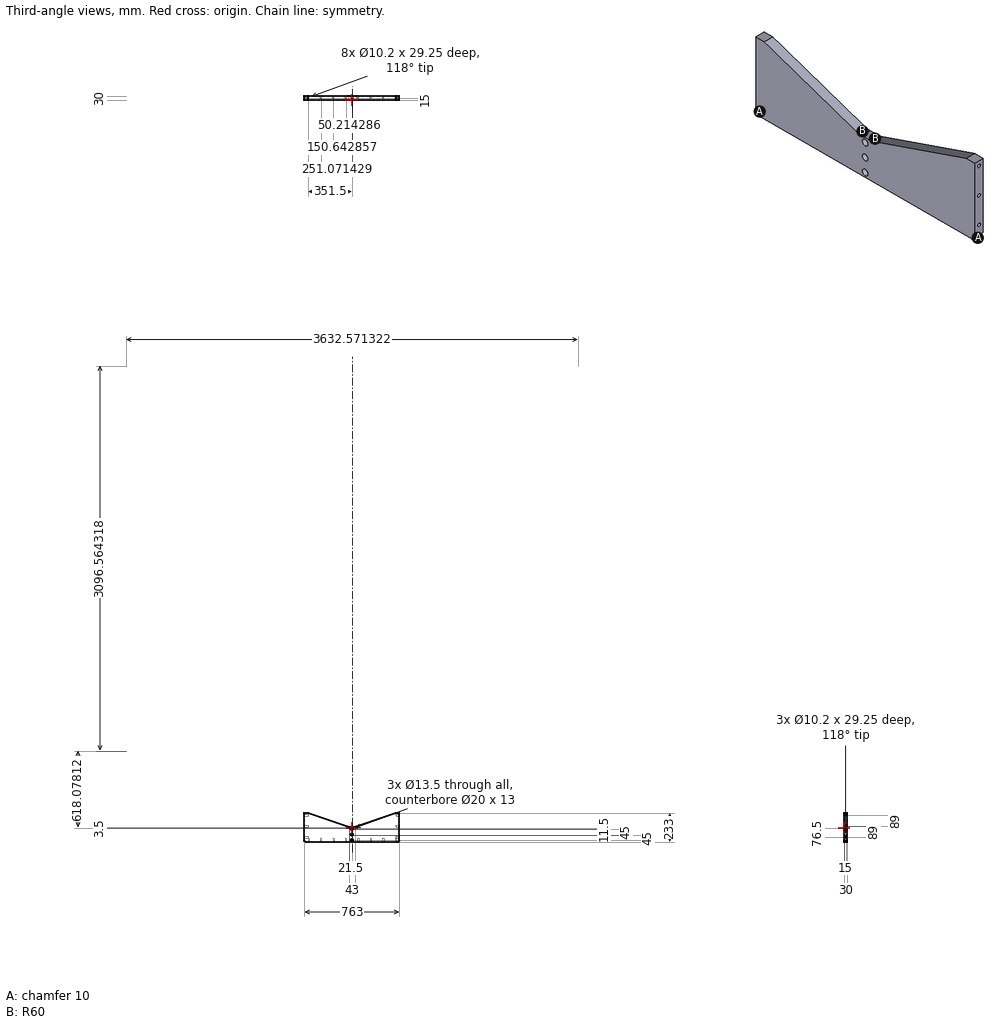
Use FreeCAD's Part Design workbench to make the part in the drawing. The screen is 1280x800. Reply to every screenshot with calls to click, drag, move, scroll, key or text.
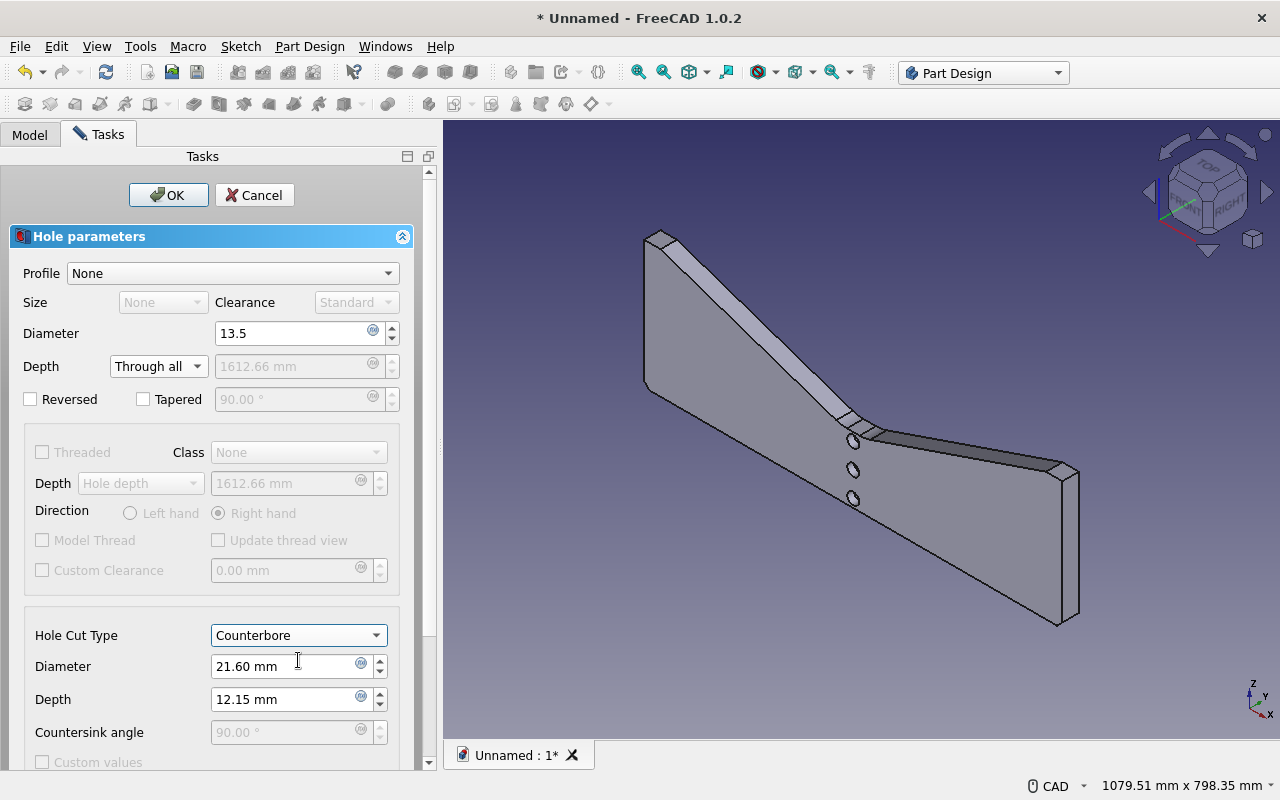
triple_click(292, 666)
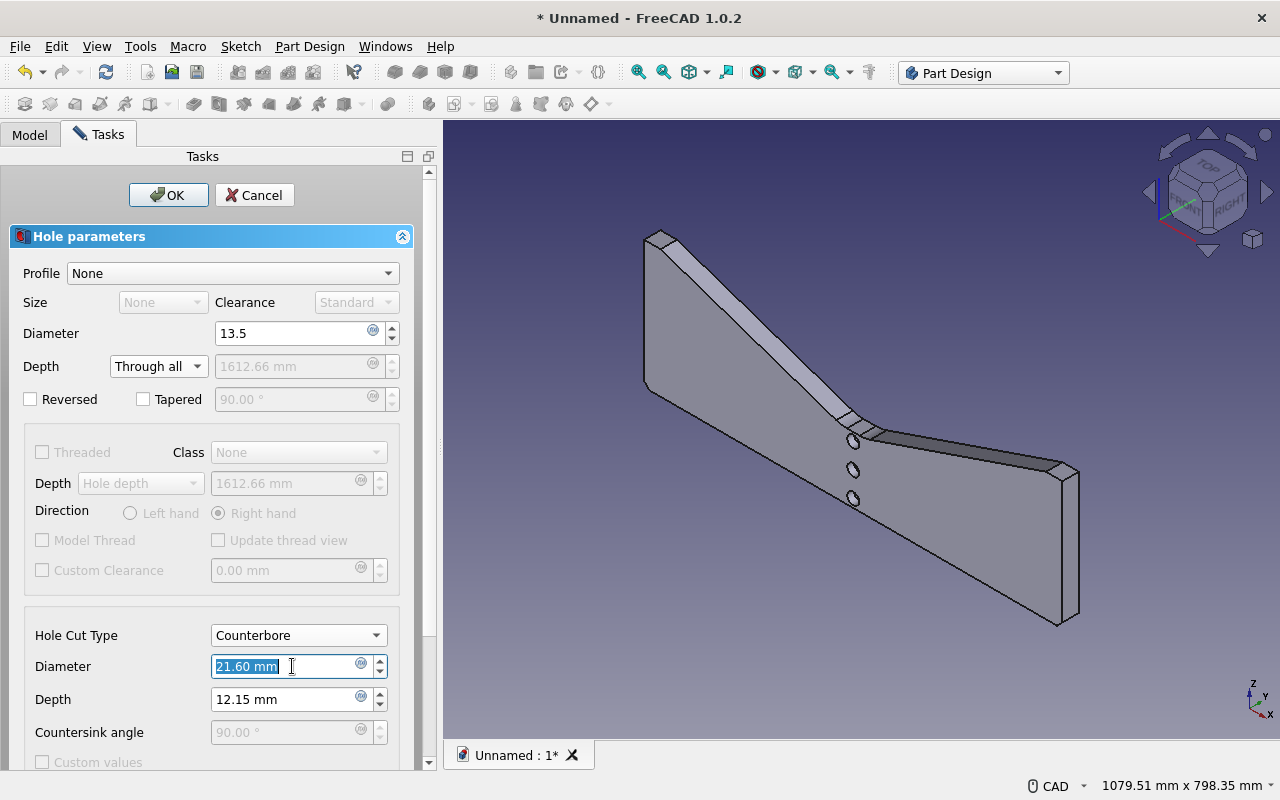
text(20)
key(Tab)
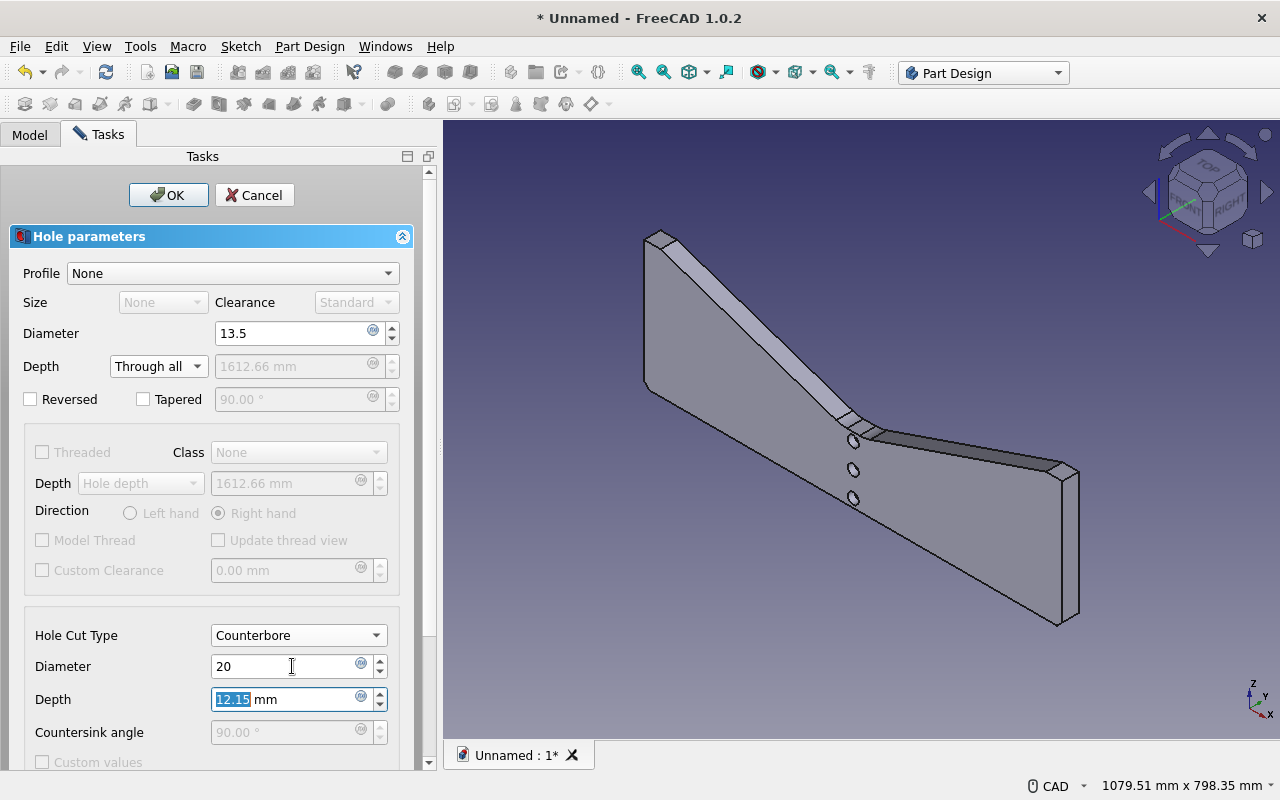
text(13)
key(Tab)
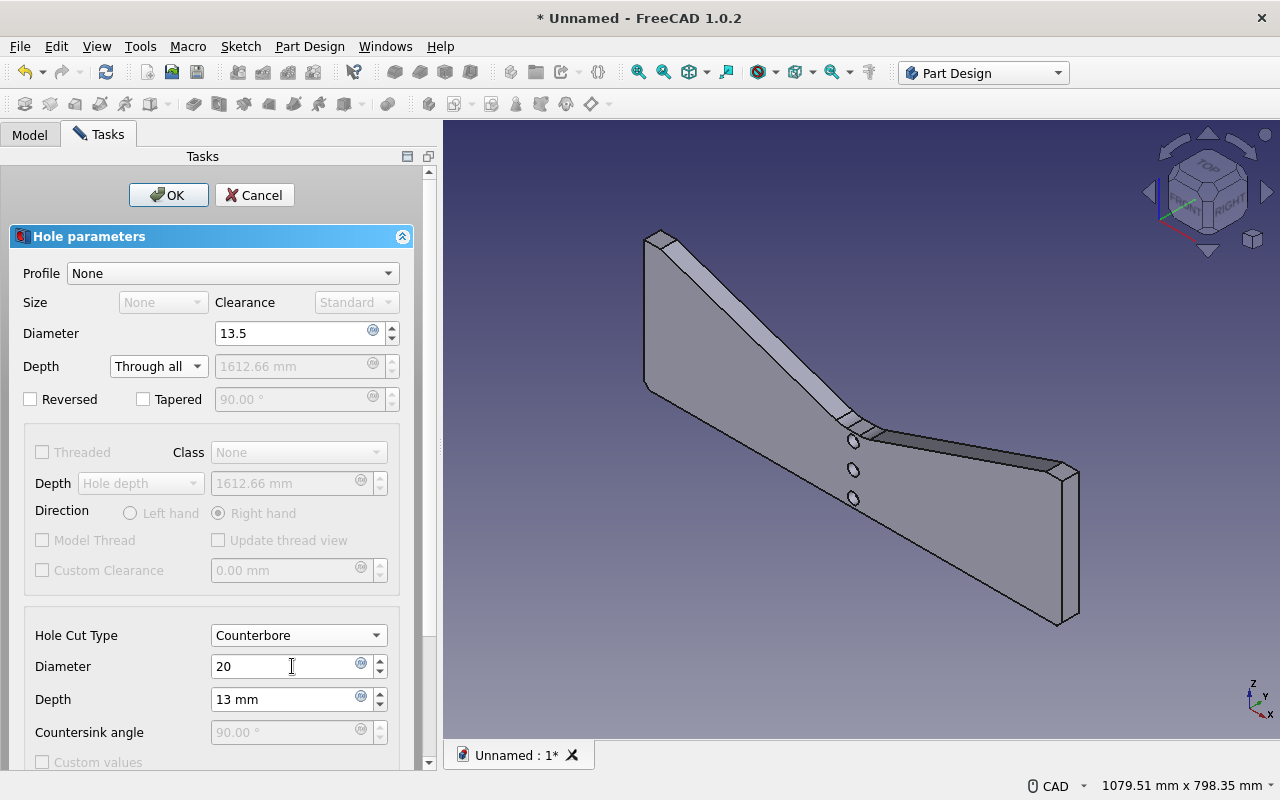
click(169, 195)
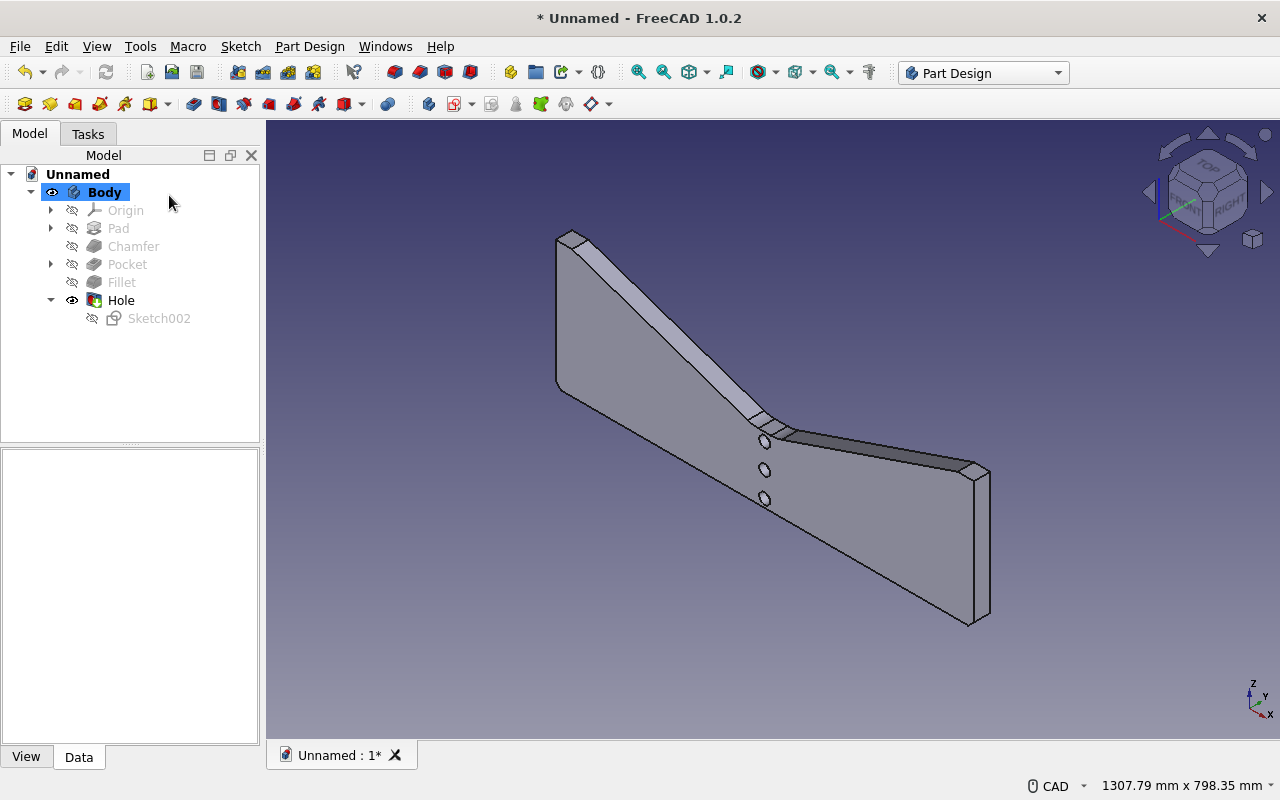
key(5)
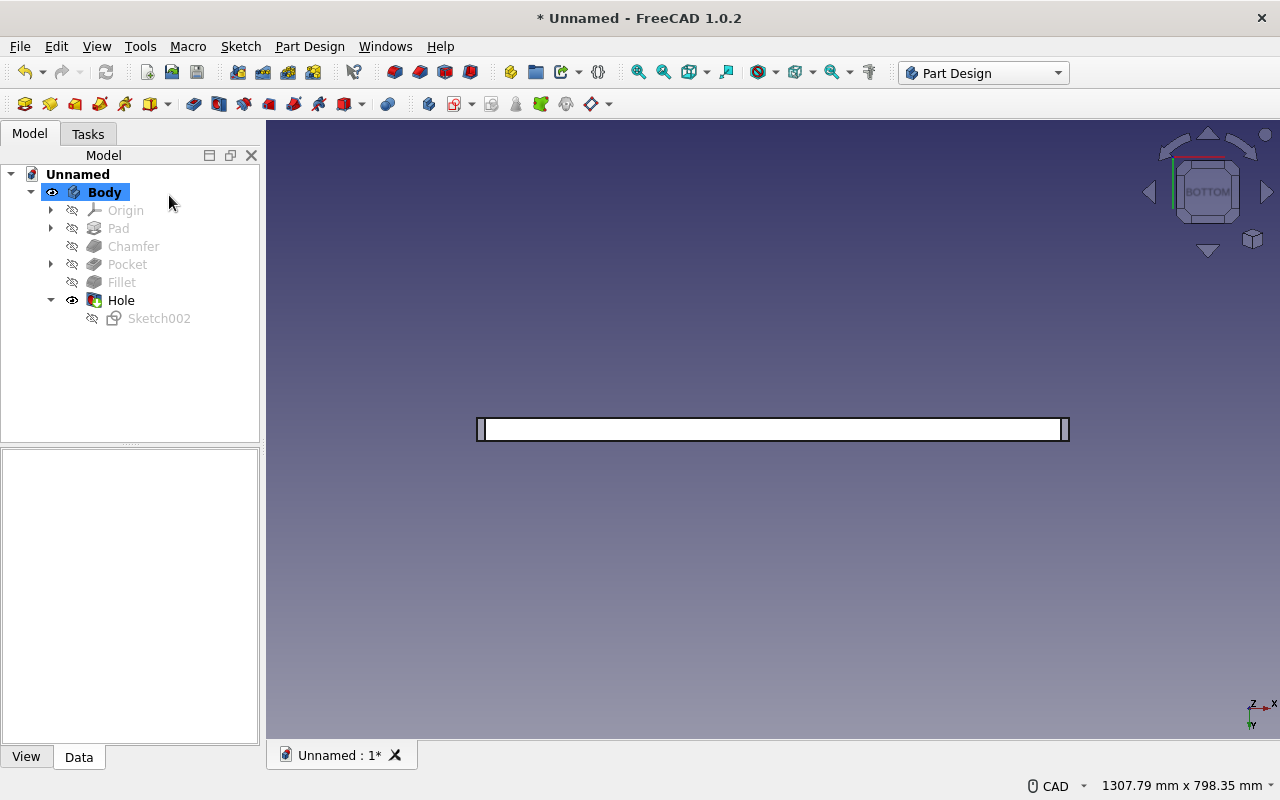
click(1020, 429)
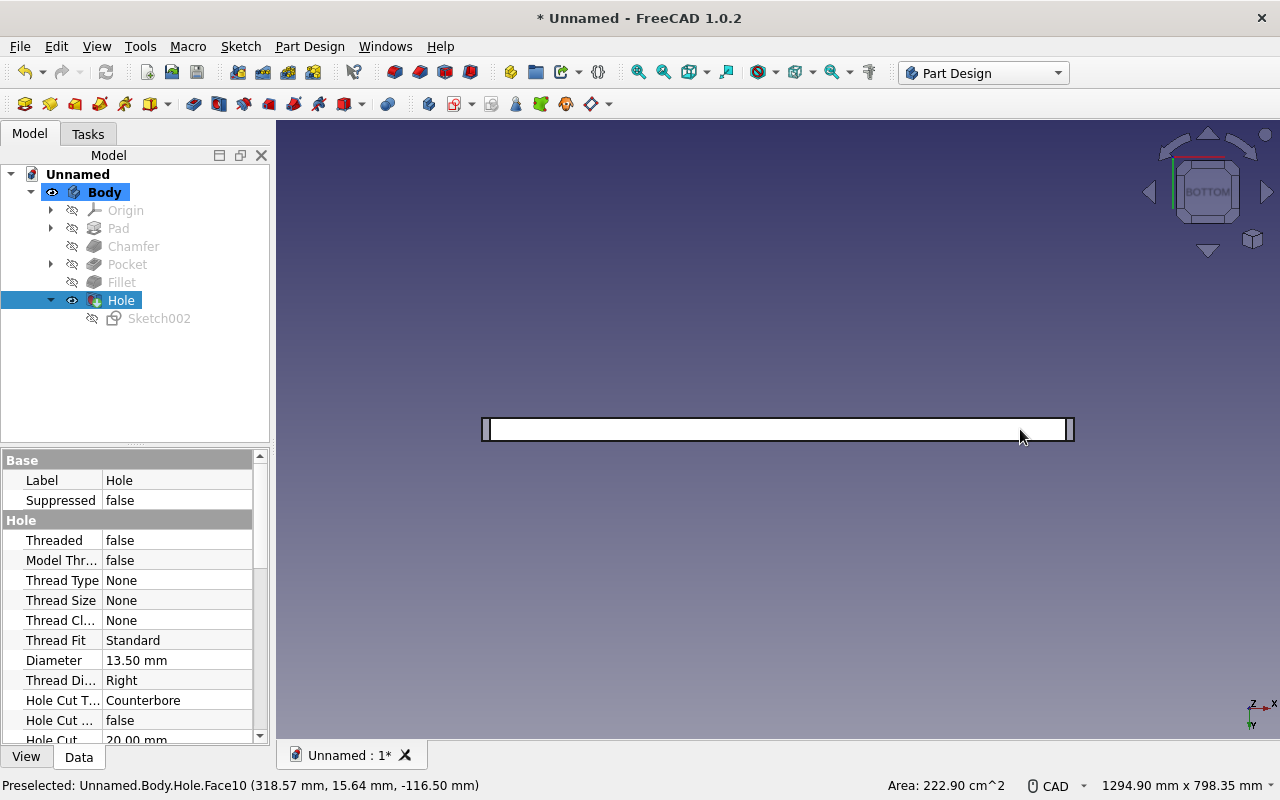
click(454, 104)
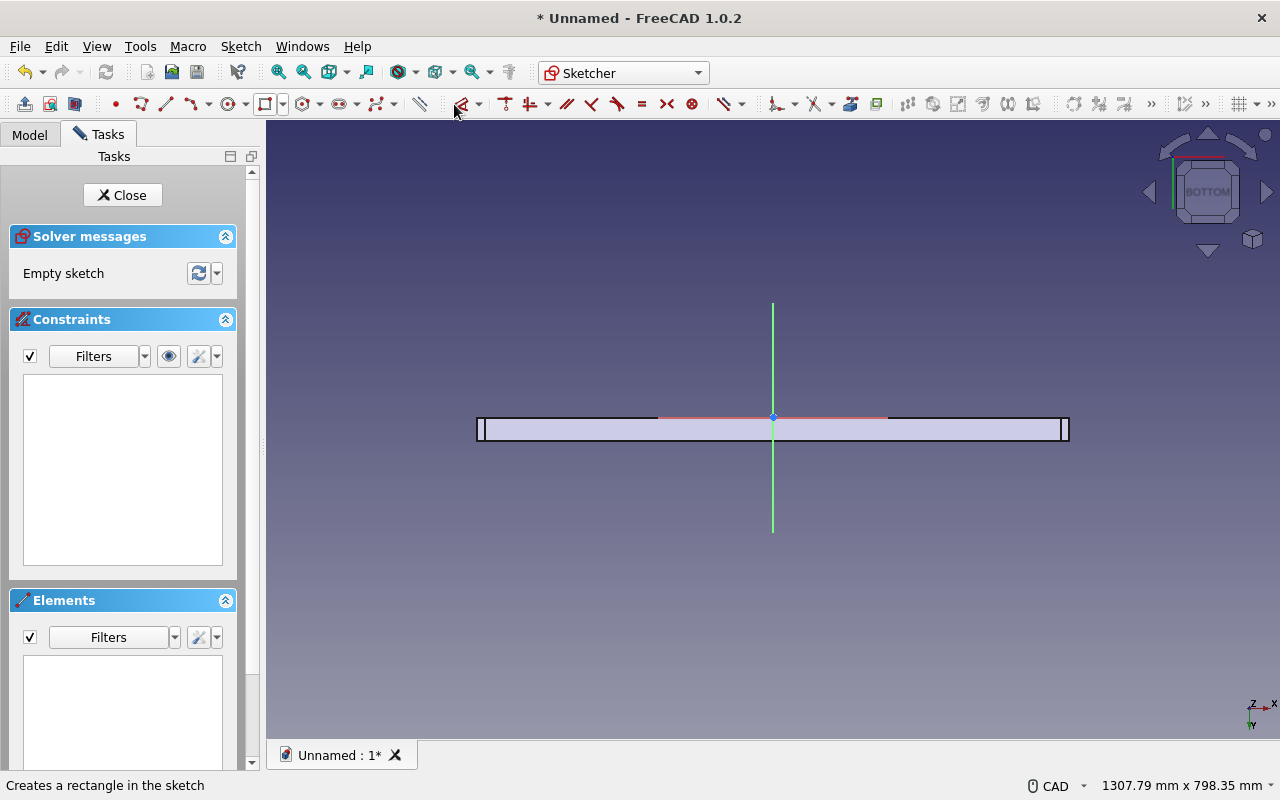
key(g)
key(c)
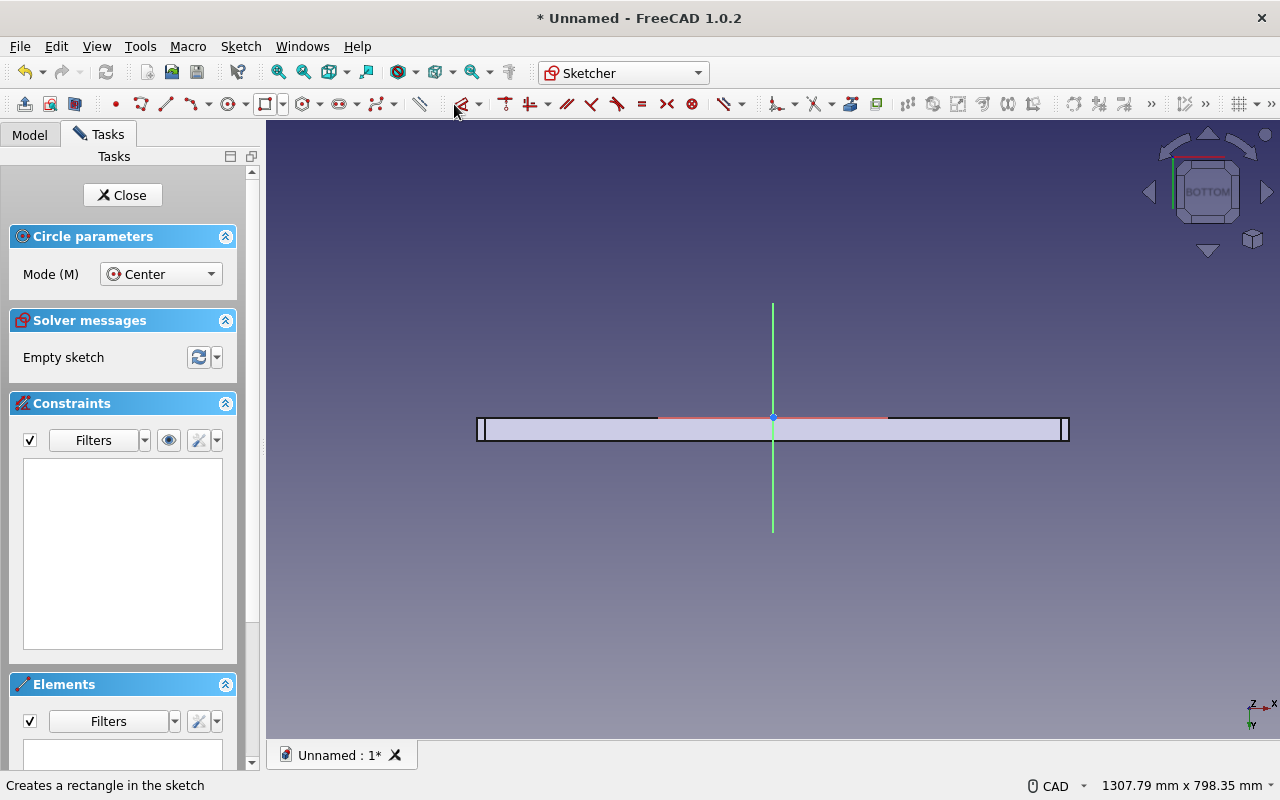
scroll(500, 430, up, 9)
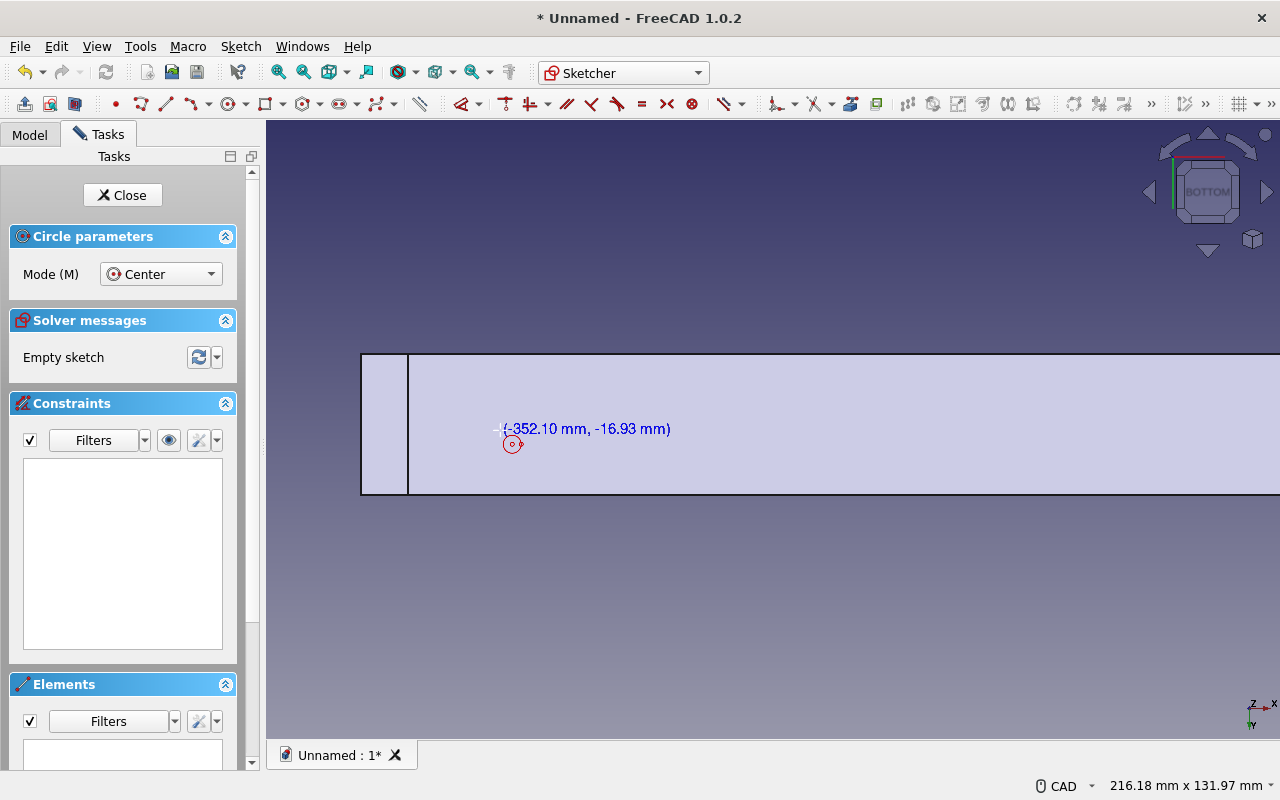
scroll(418, 435, down, 9)